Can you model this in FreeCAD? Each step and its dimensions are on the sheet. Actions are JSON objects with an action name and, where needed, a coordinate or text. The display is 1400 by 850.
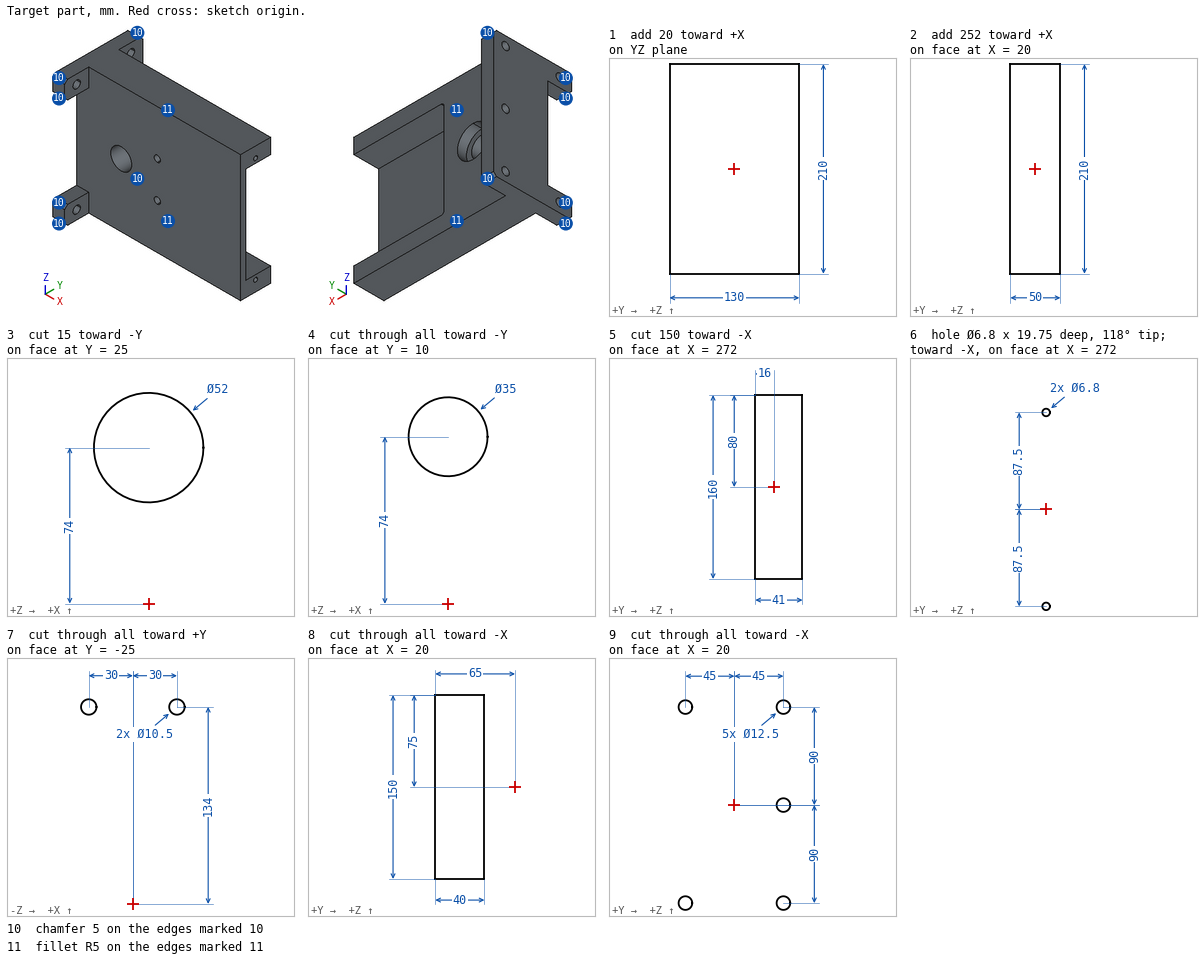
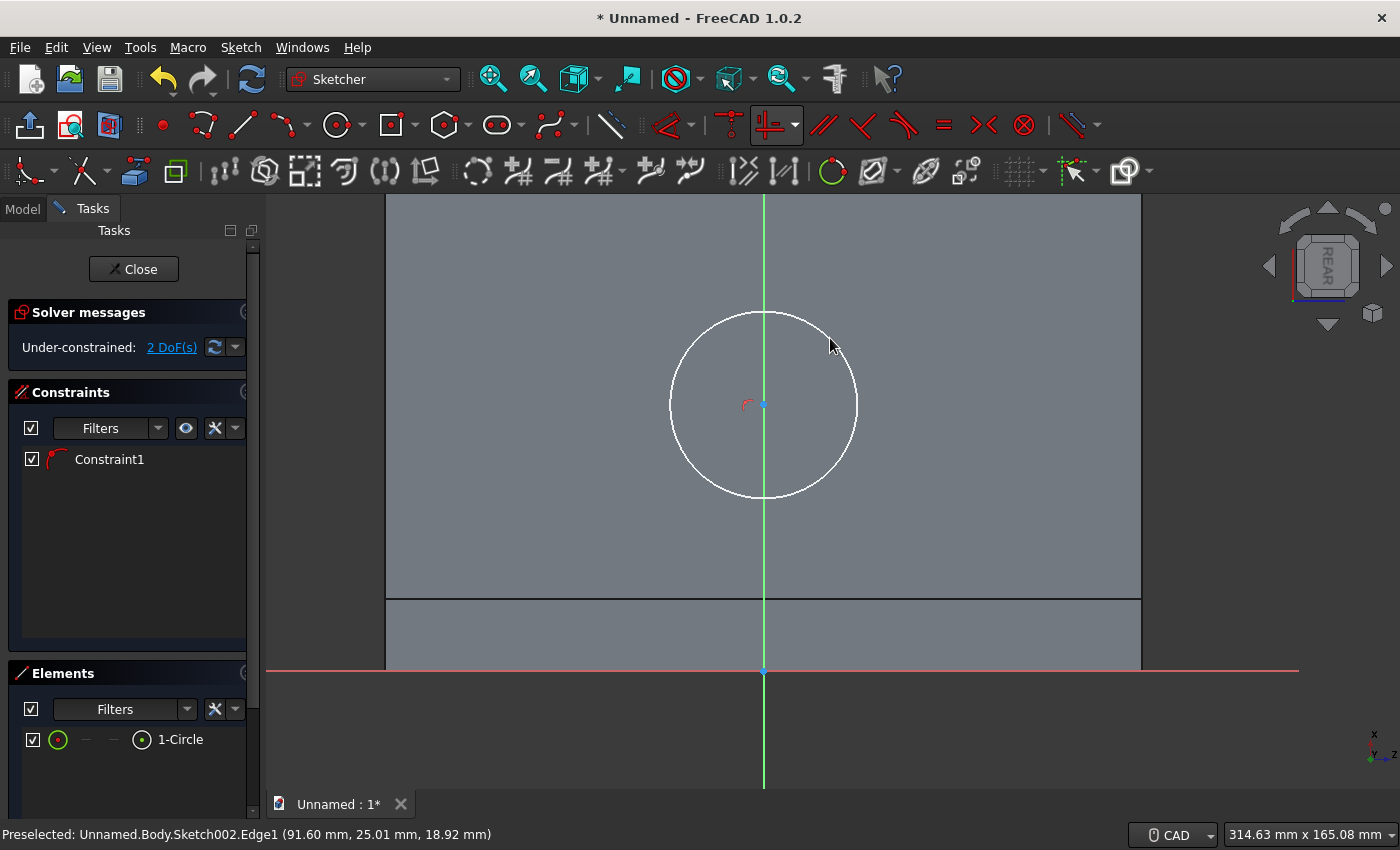
{"action": "left_click", "coordinate": [666, 126]}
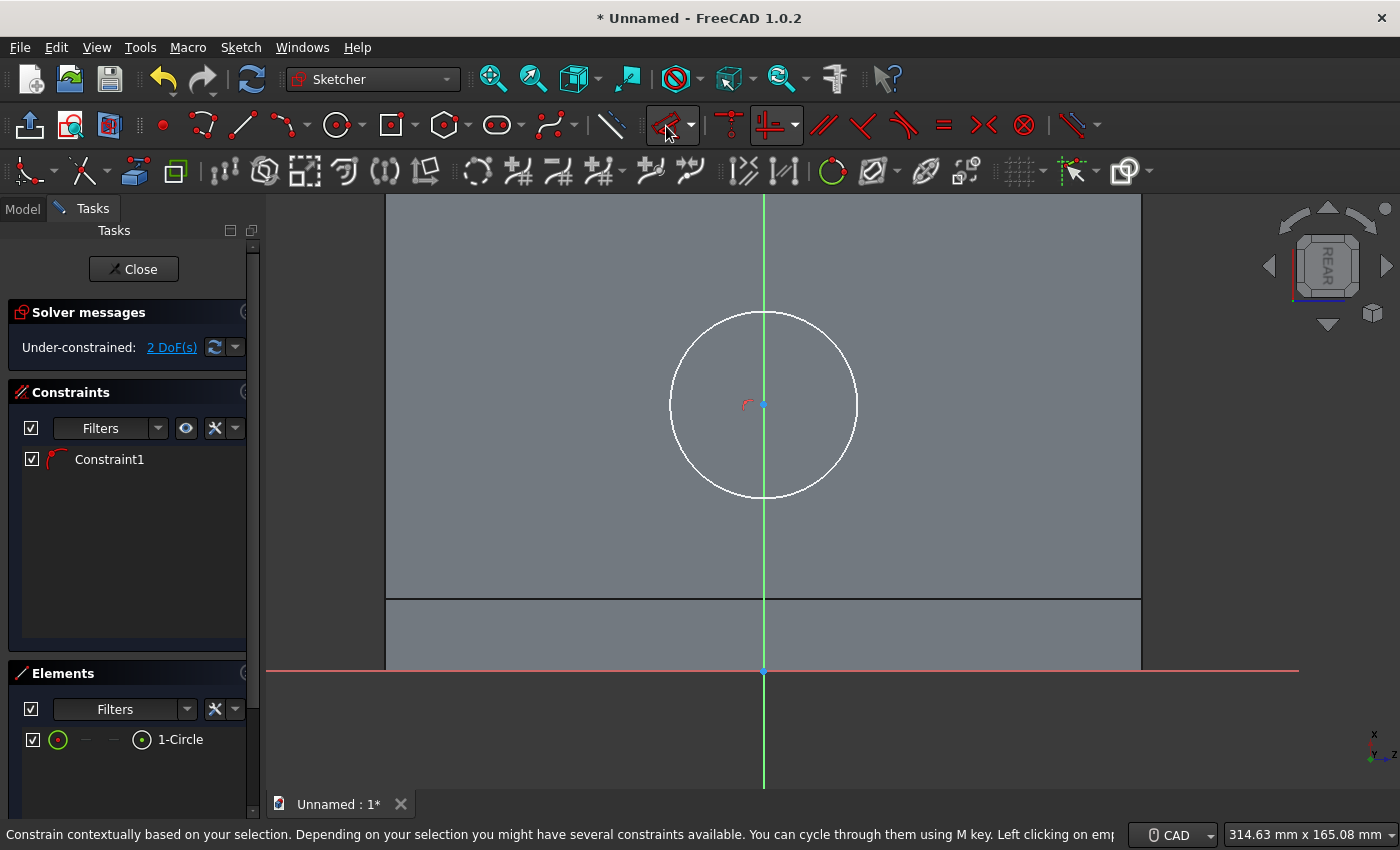
{"action": "left_click", "coordinate": [830, 339]}
{"action": "left_click", "coordinate": [853, 316]}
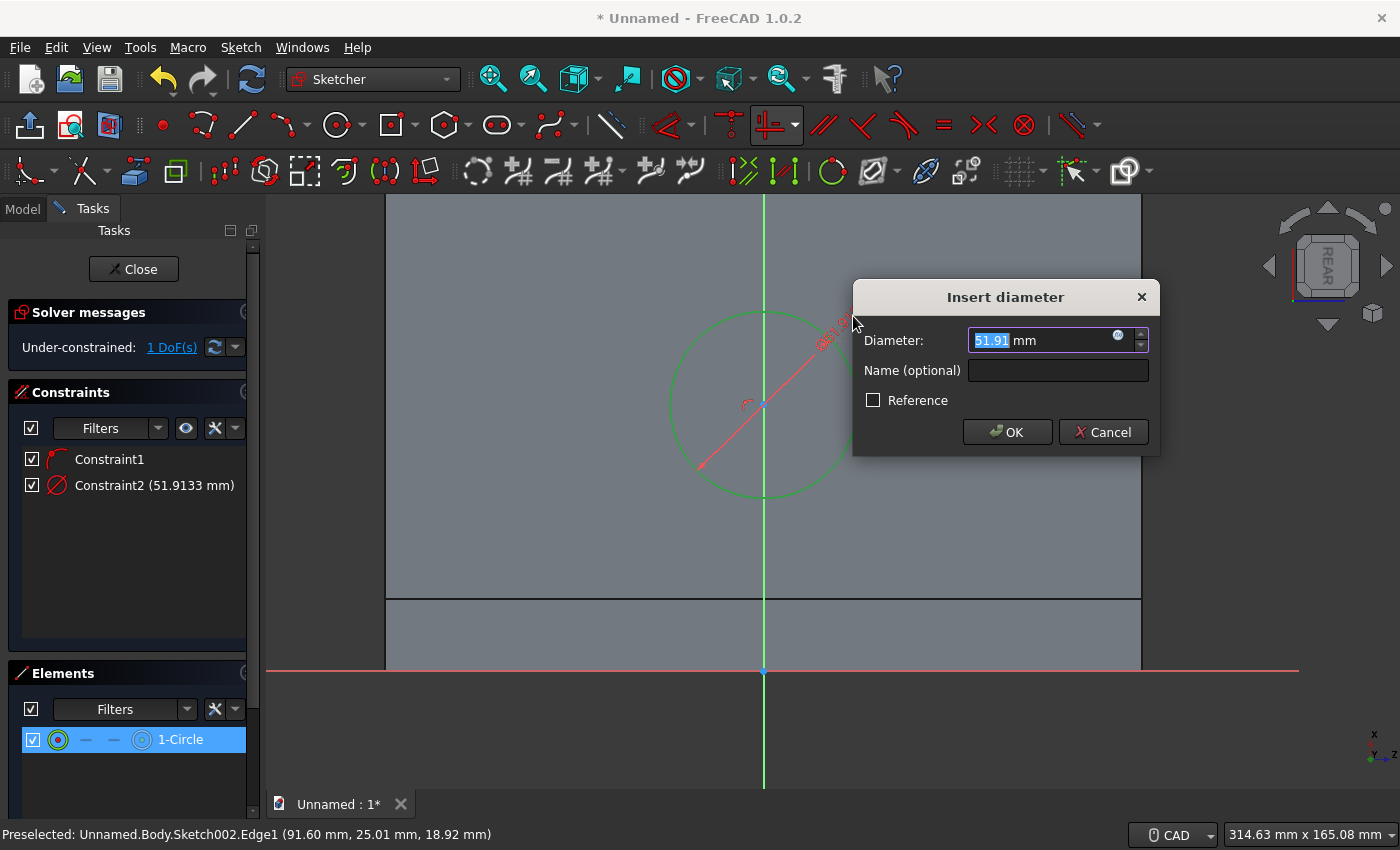
{"action": "type", "text": "52"}
{"action": "key", "text": "Return"}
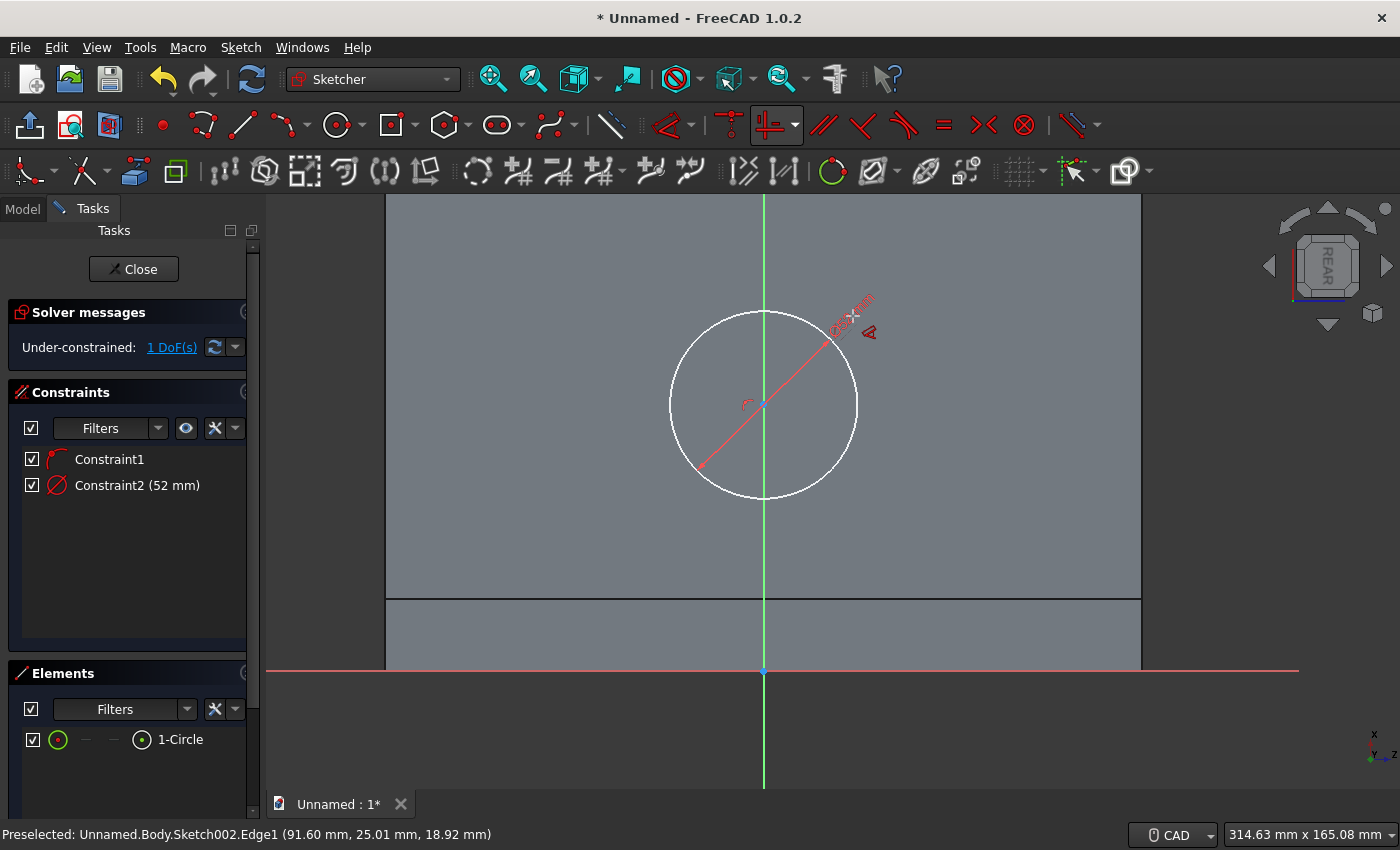
{"action": "left_click", "coordinate": [764, 405]}
{"action": "left_click", "coordinate": [798, 538]}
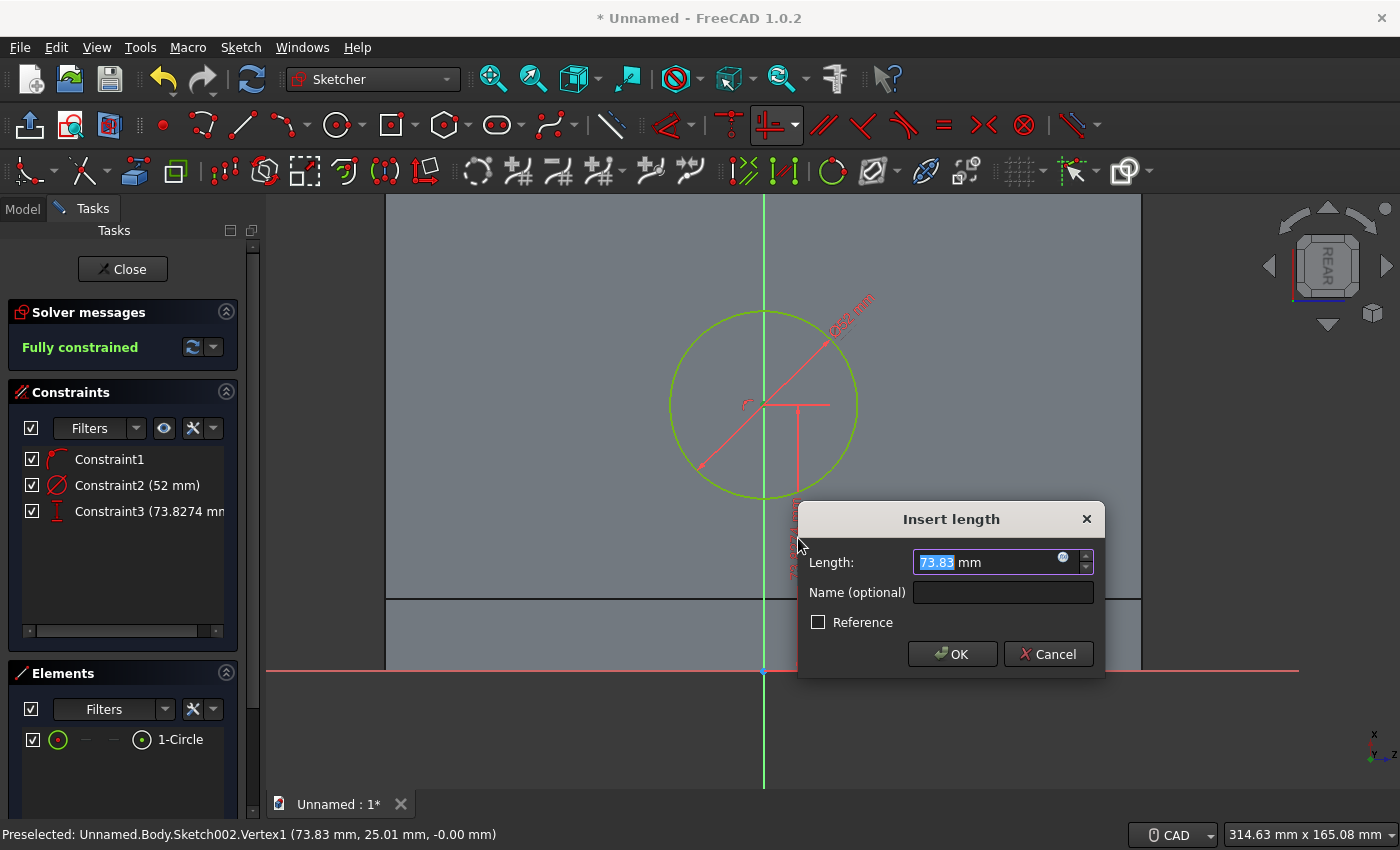
{"action": "type", "text": "74"}
{"action": "key", "text": "Return"}
{"action": "key", "text": "Escape"}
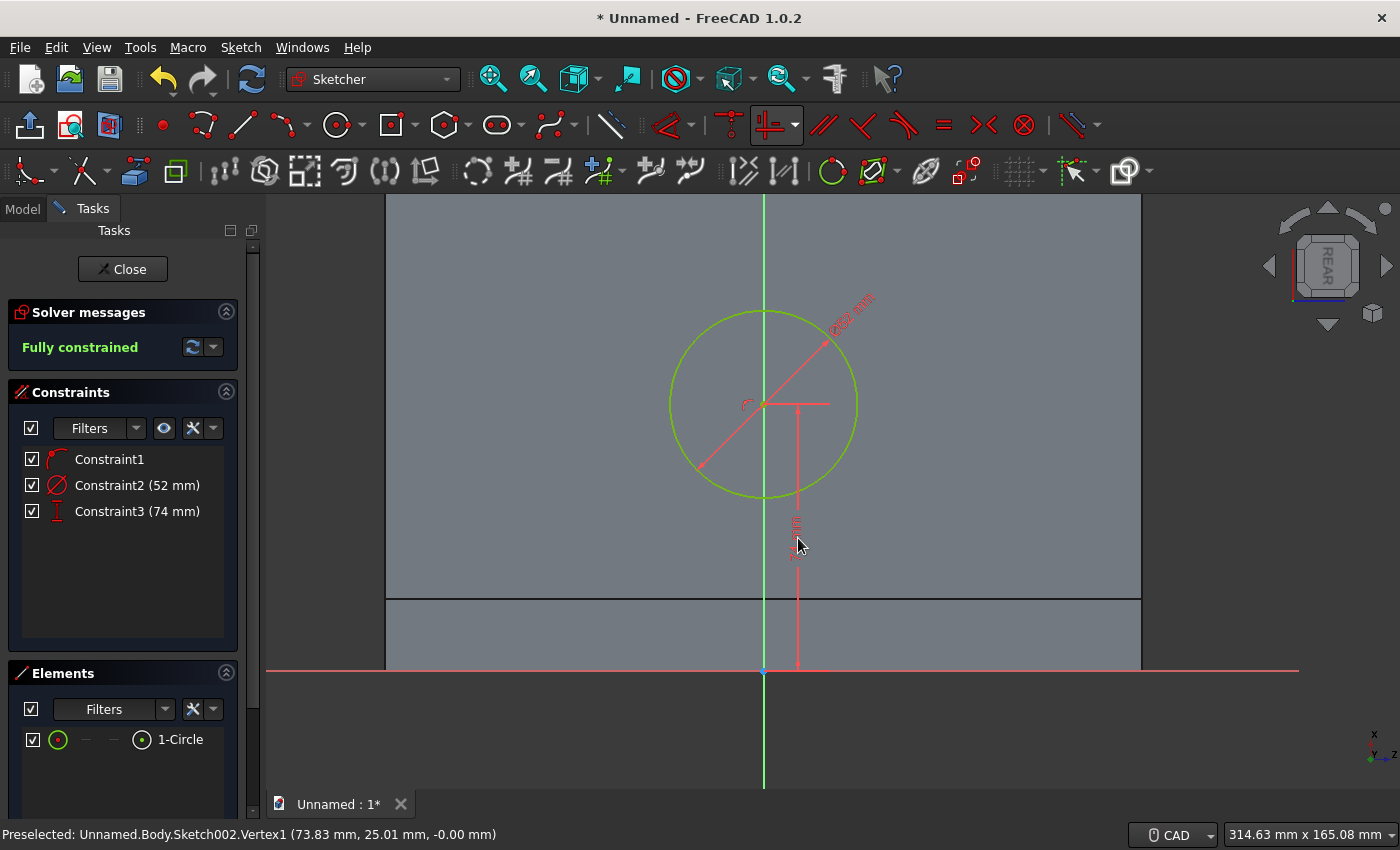
{"action": "left_click", "coordinate": [123, 269]}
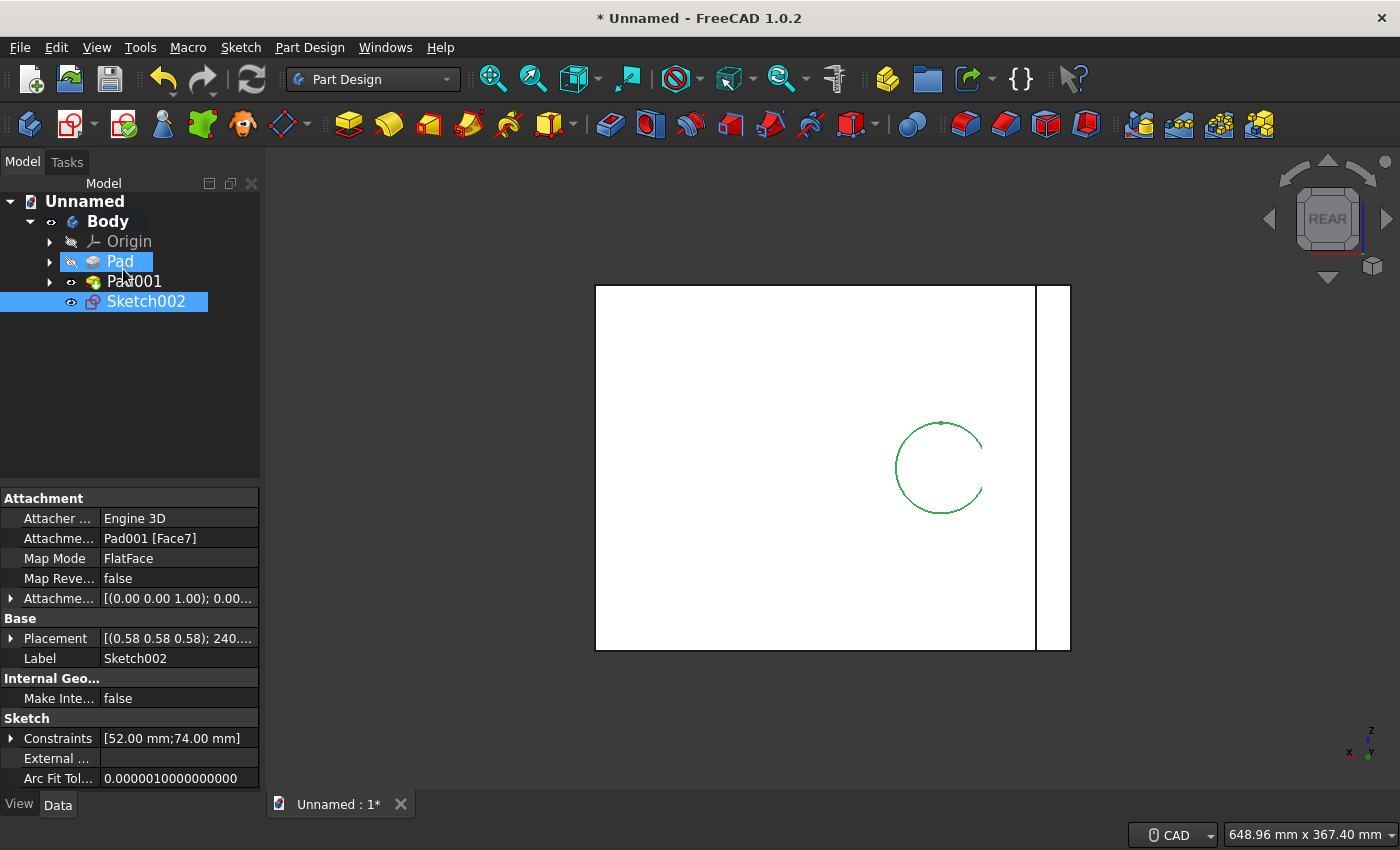
{"action": "left_click", "coordinate": [612, 124]}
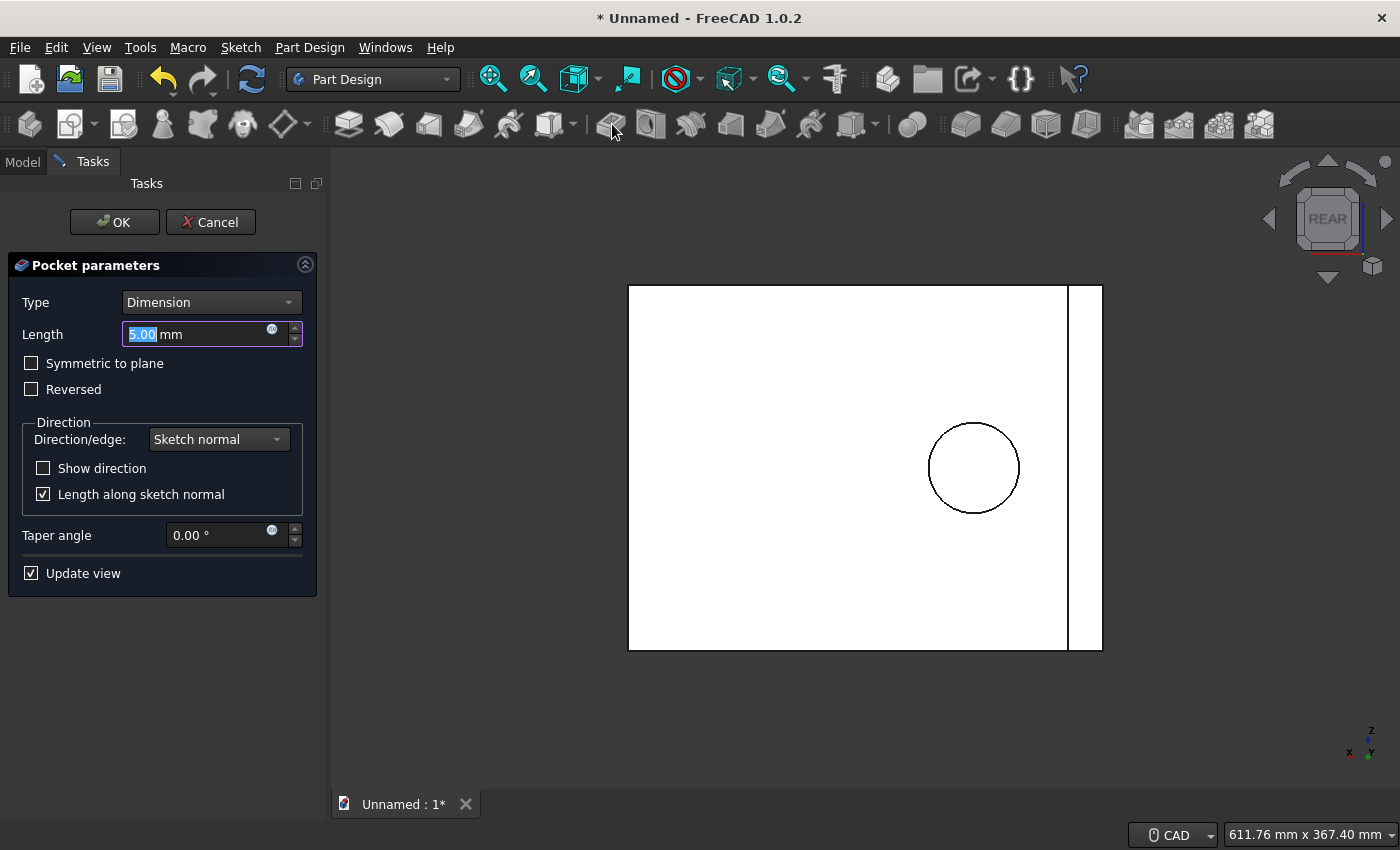
{"action": "type", "text": "15"}
{"action": "key", "text": "Tab"}